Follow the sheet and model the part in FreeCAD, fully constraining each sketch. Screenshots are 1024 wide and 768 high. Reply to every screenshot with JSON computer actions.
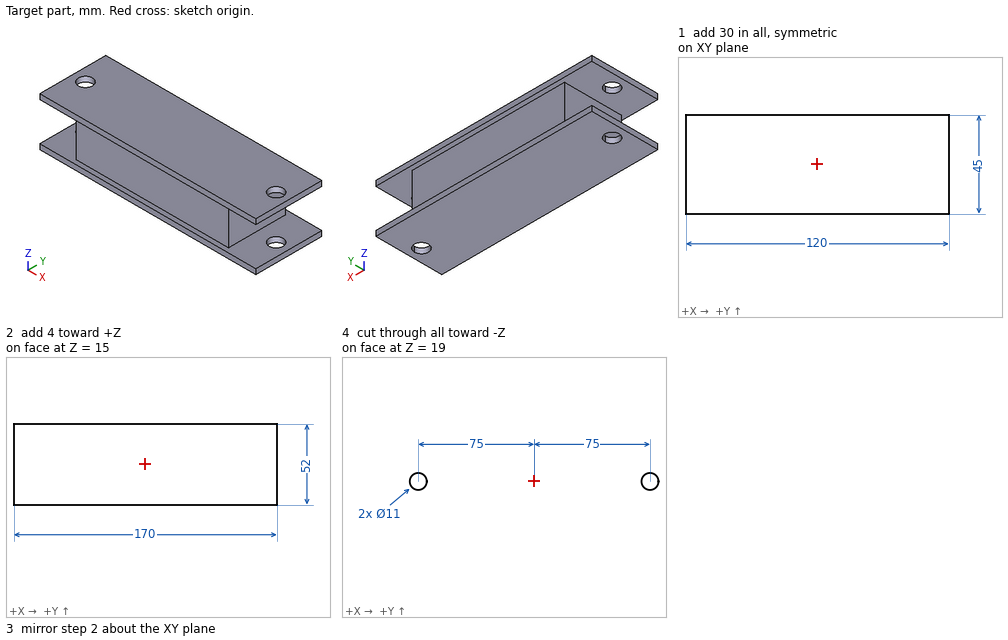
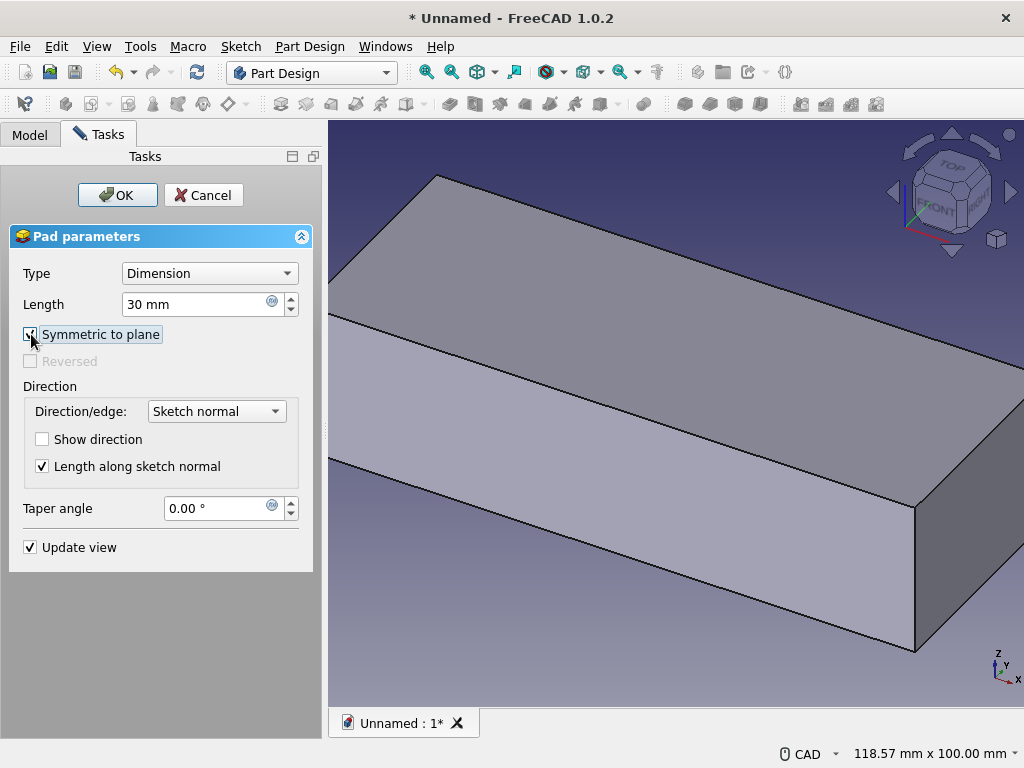
{"action": "left_click", "coordinate": [118, 195]}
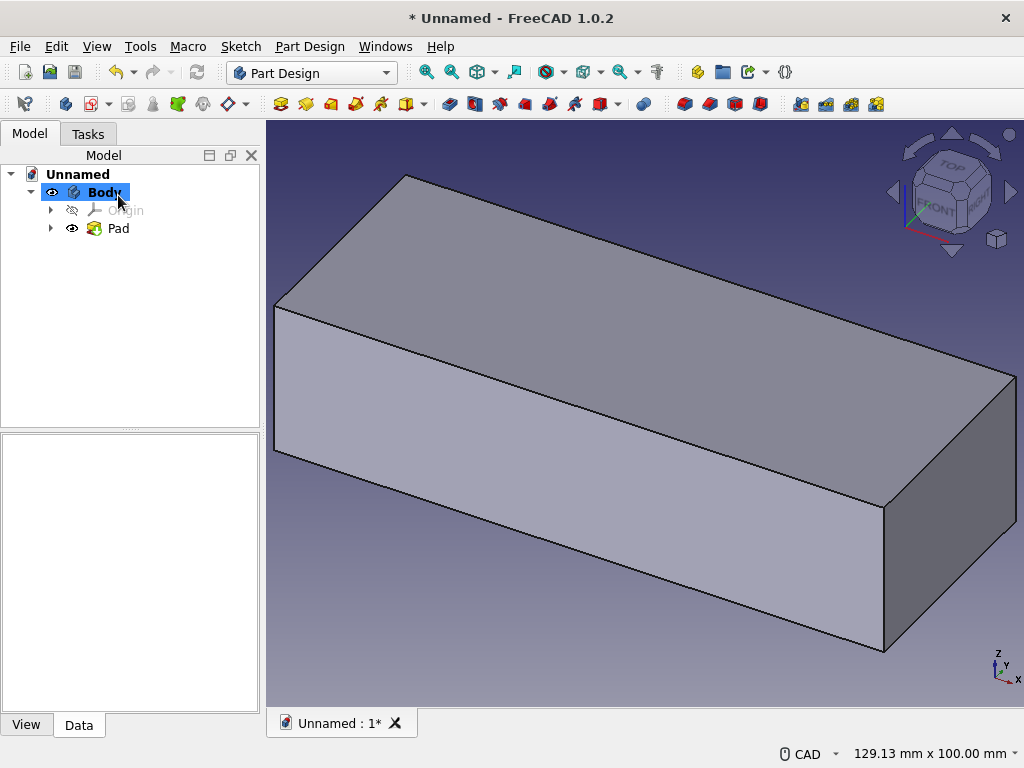
{"action": "left_click", "coordinate": [819, 398]}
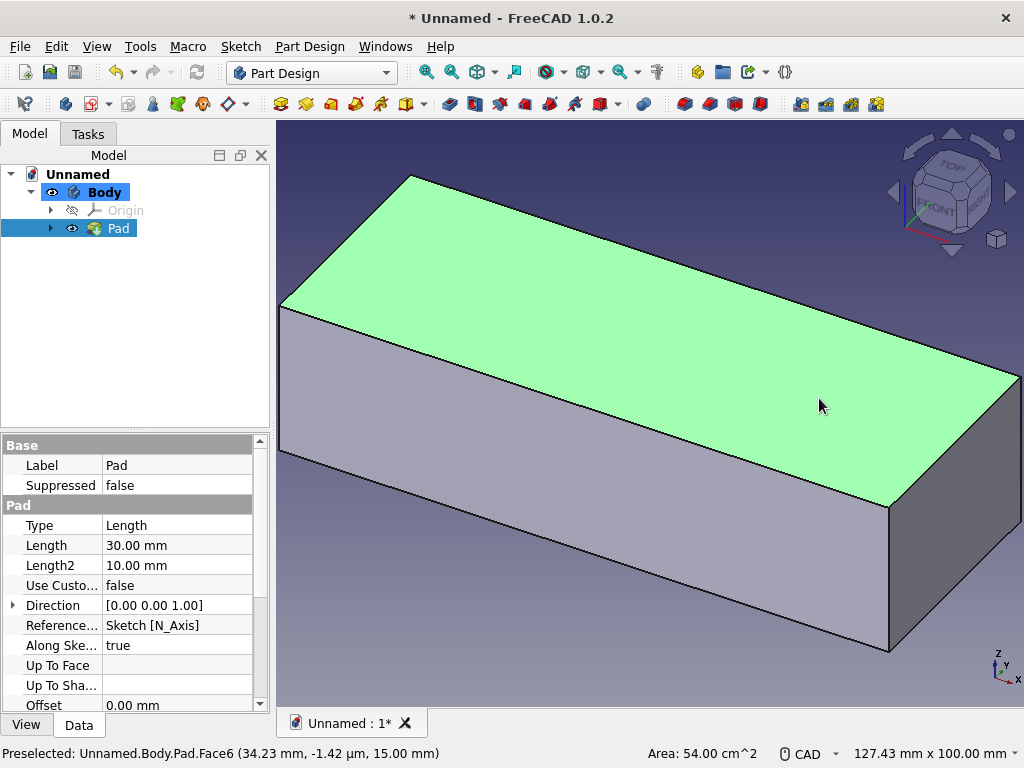
{"action": "left_click", "coordinate": [90, 104]}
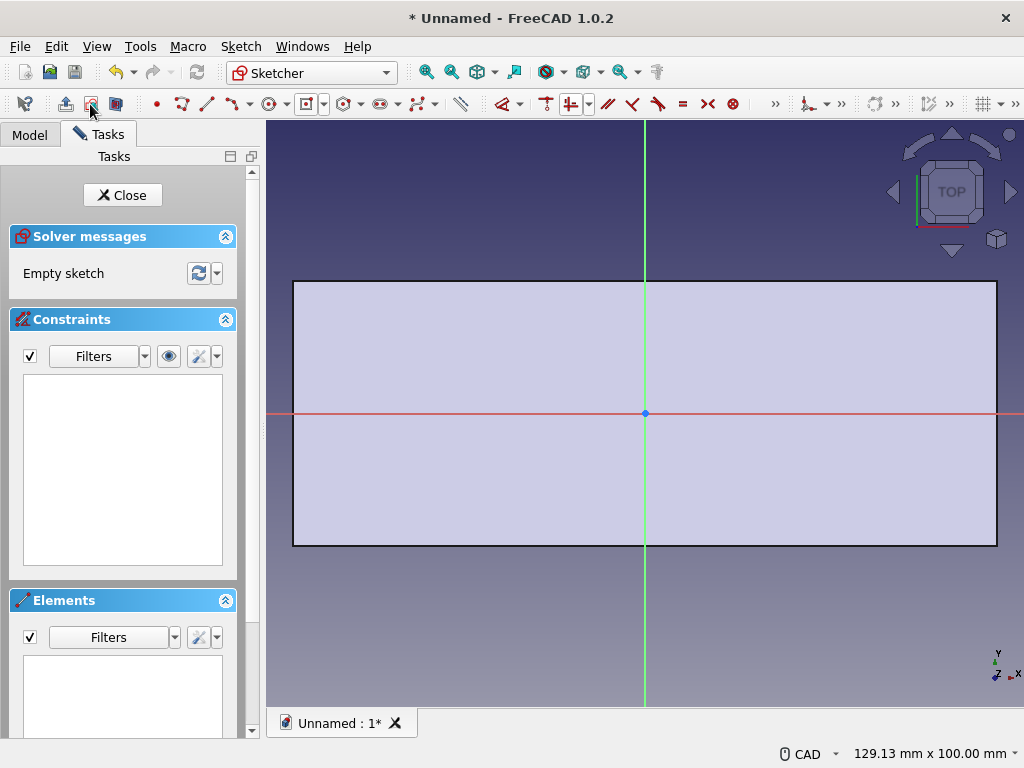
{"action": "scroll", "coordinate": [537, 414], "scroll_direction": "down", "scroll_amount": 5}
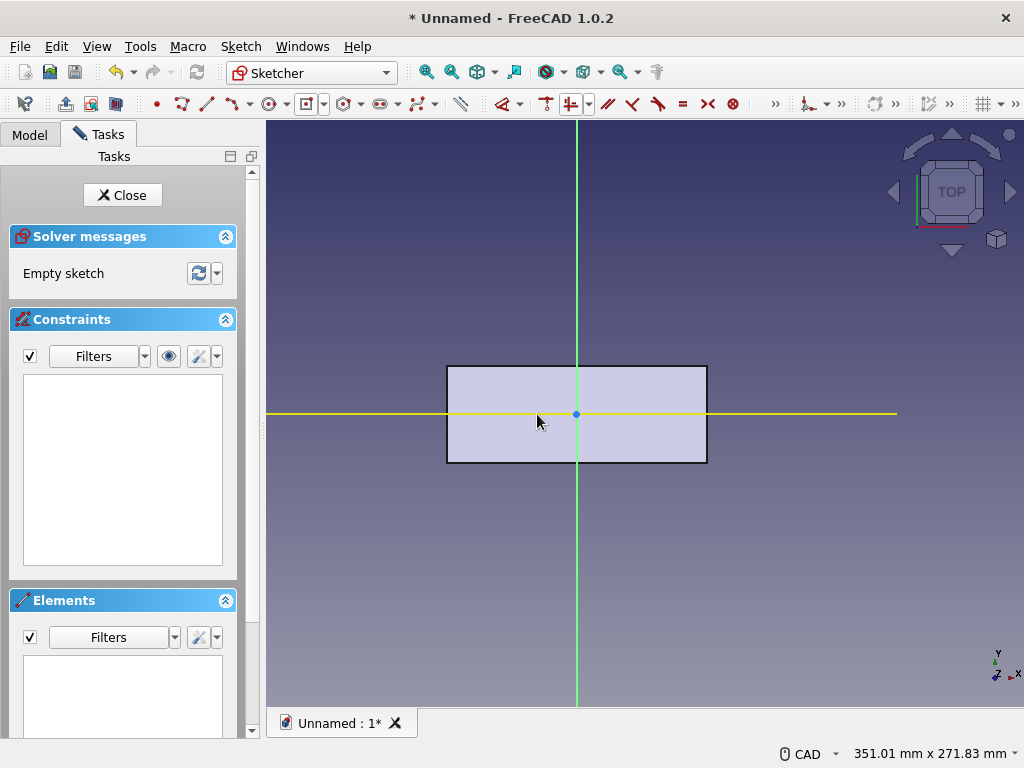
{"action": "left_click", "coordinate": [306, 104]}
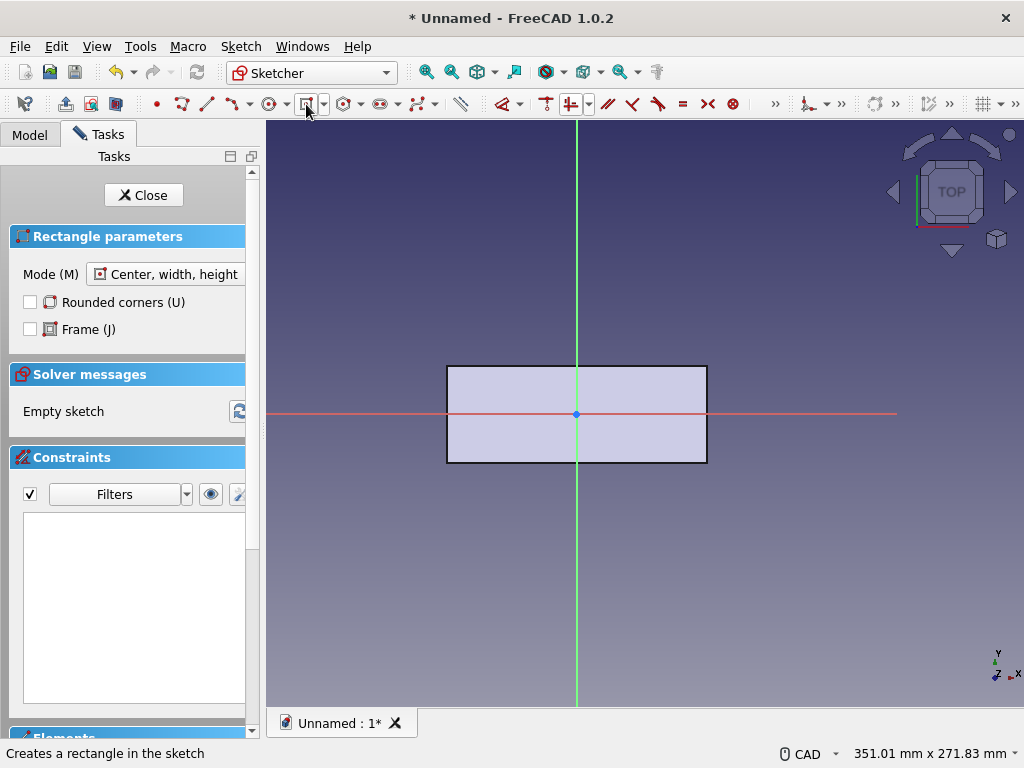
{"action": "left_click", "coordinate": [577, 414]}
{"action": "mouse_move", "coordinate": [761, 358]}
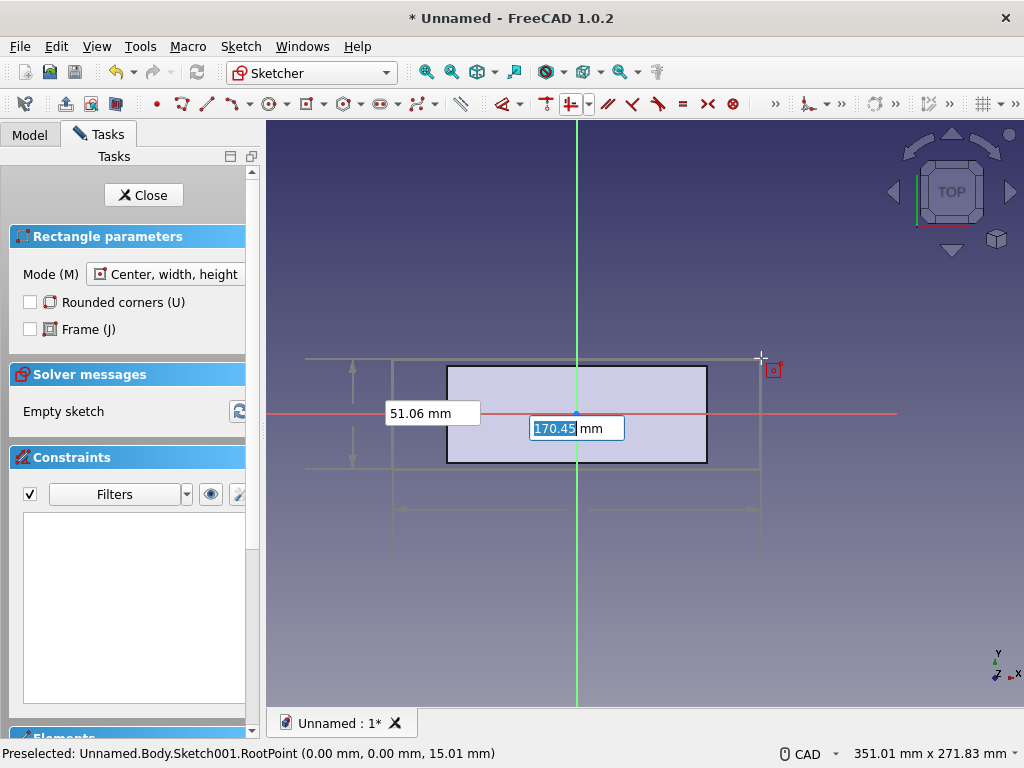
{"action": "type", "text": "170"}
{"action": "key", "text": "Tab"}
{"action": "type", "text": "52"}
{"action": "key", "text": "Return"}
{"action": "key", "text": "Escape"}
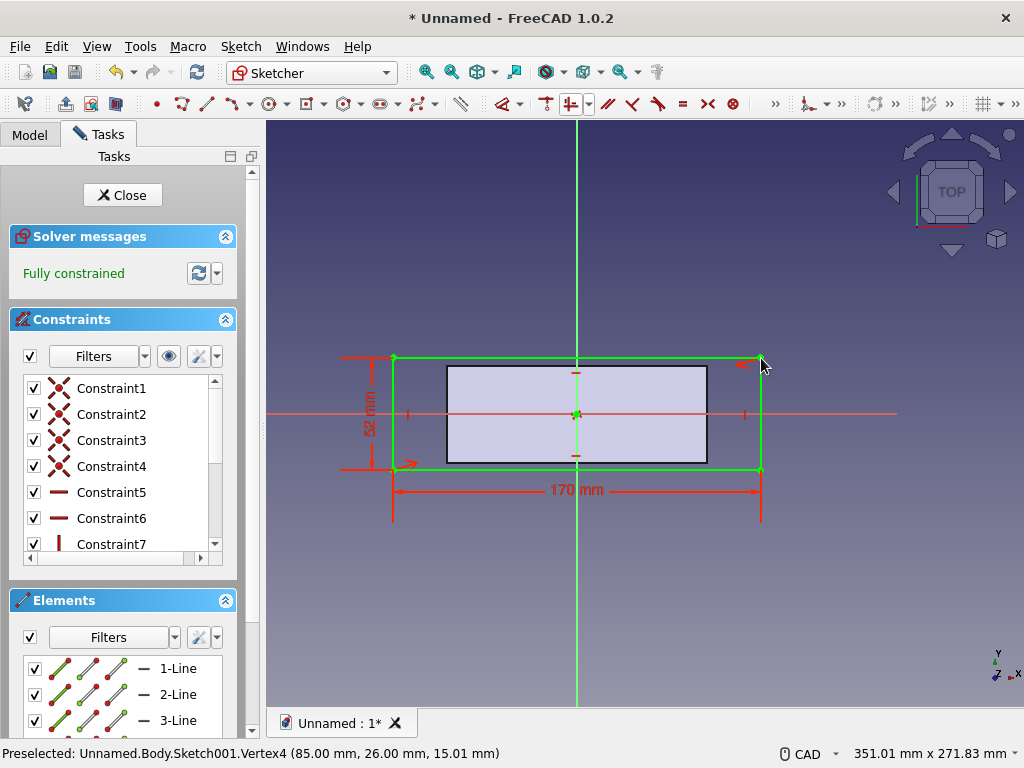
{"action": "left_click", "coordinate": [123, 195]}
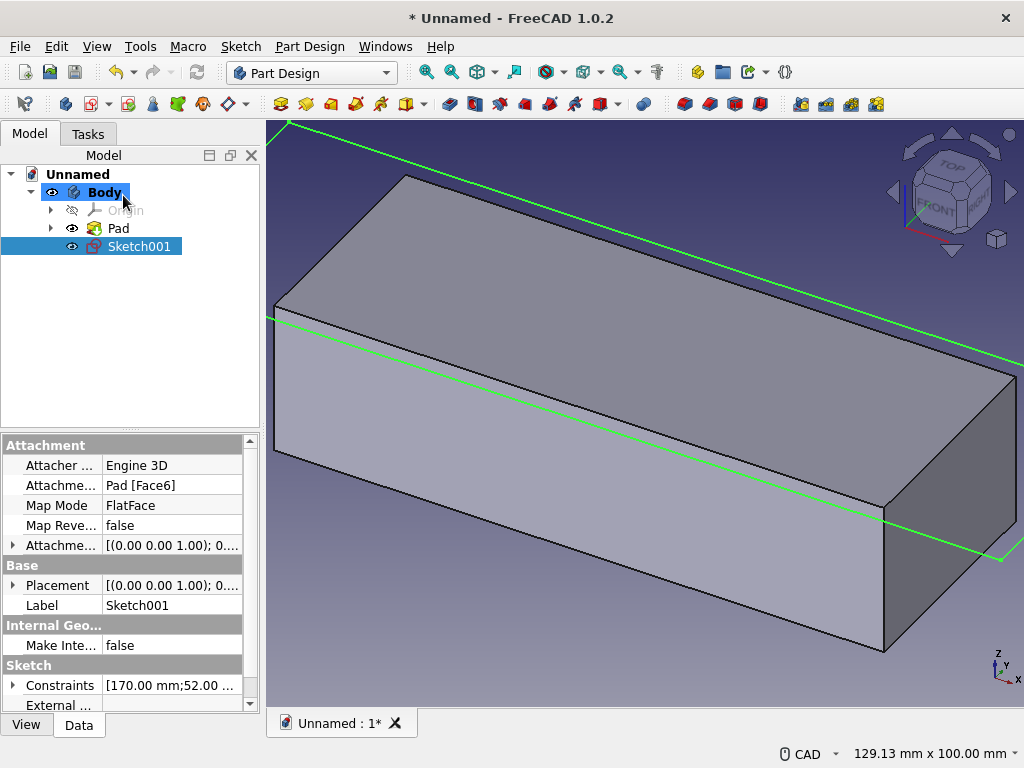
{"action": "left_click", "coordinate": [281, 104]}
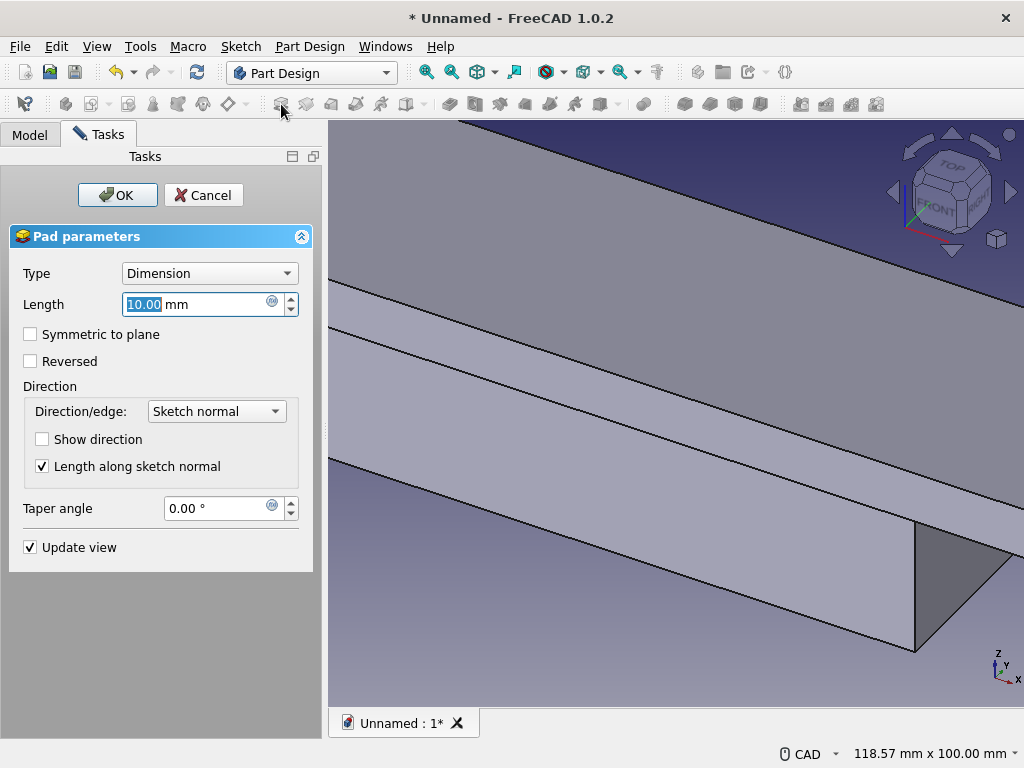
{"action": "type", "text": "4"}
{"action": "key", "text": "Tab"}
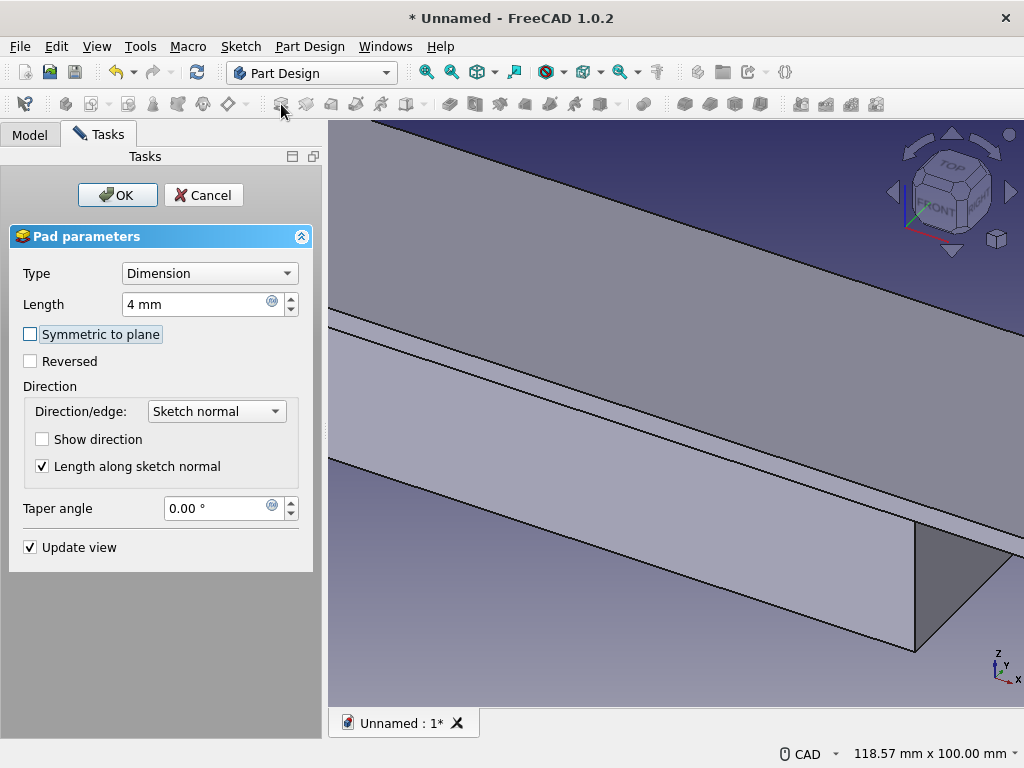
{"action": "left_click", "coordinate": [118, 195]}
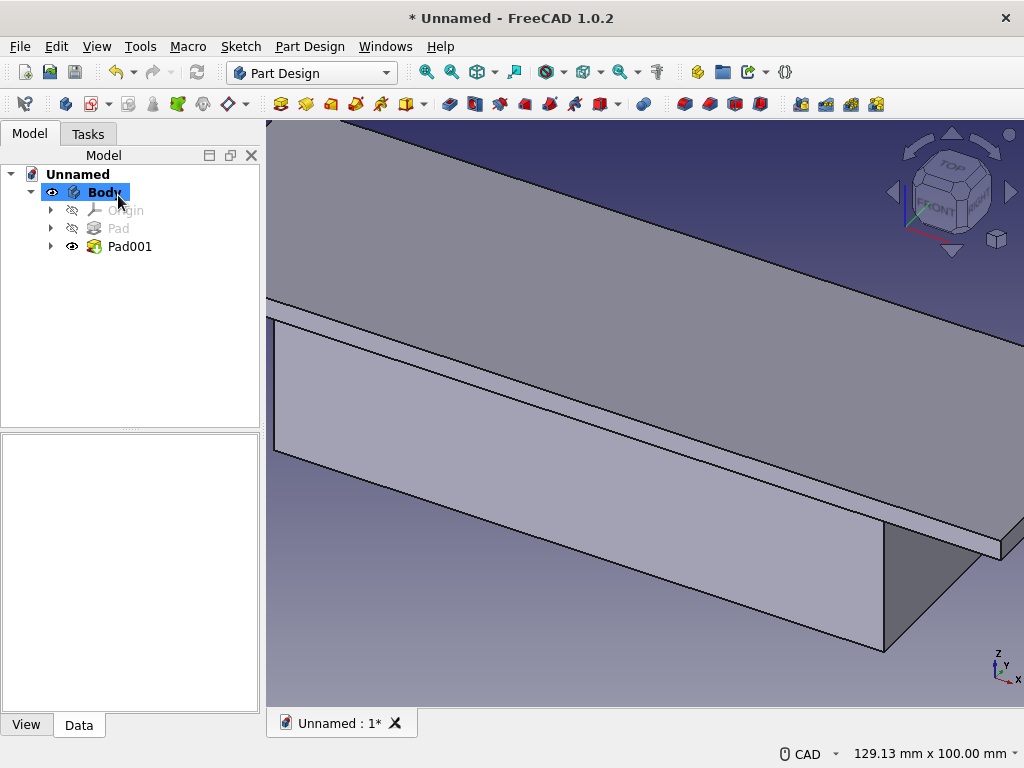
{"action": "left_click", "coordinate": [427, 72]}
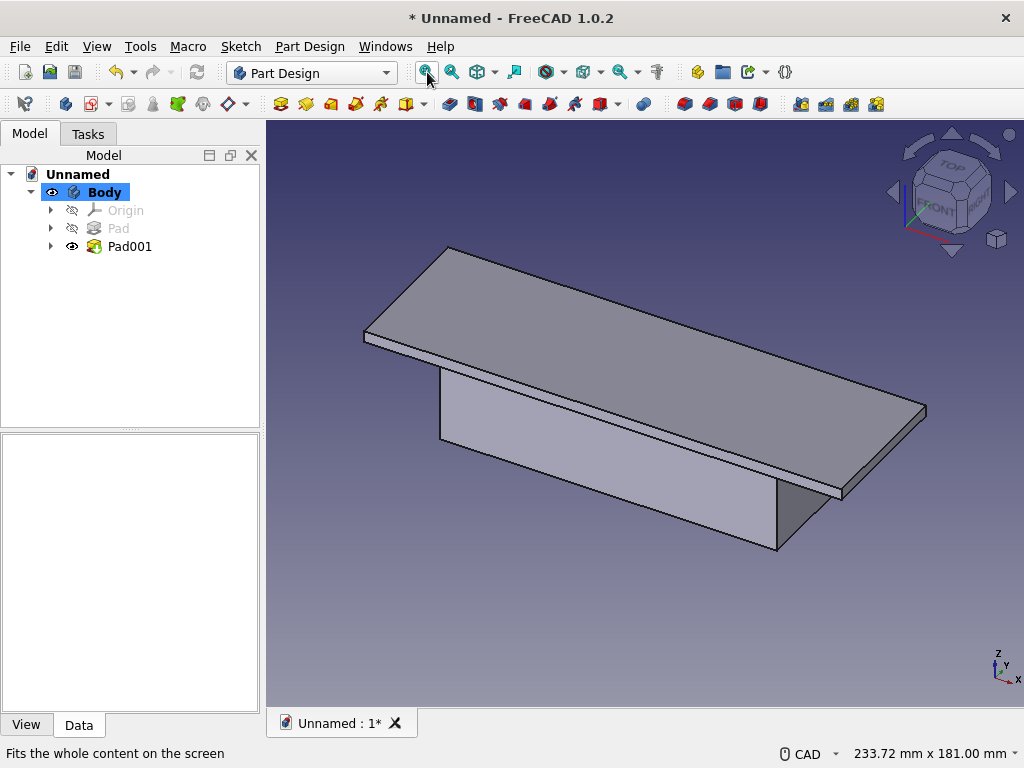
{"action": "left_click", "coordinate": [117, 246]}